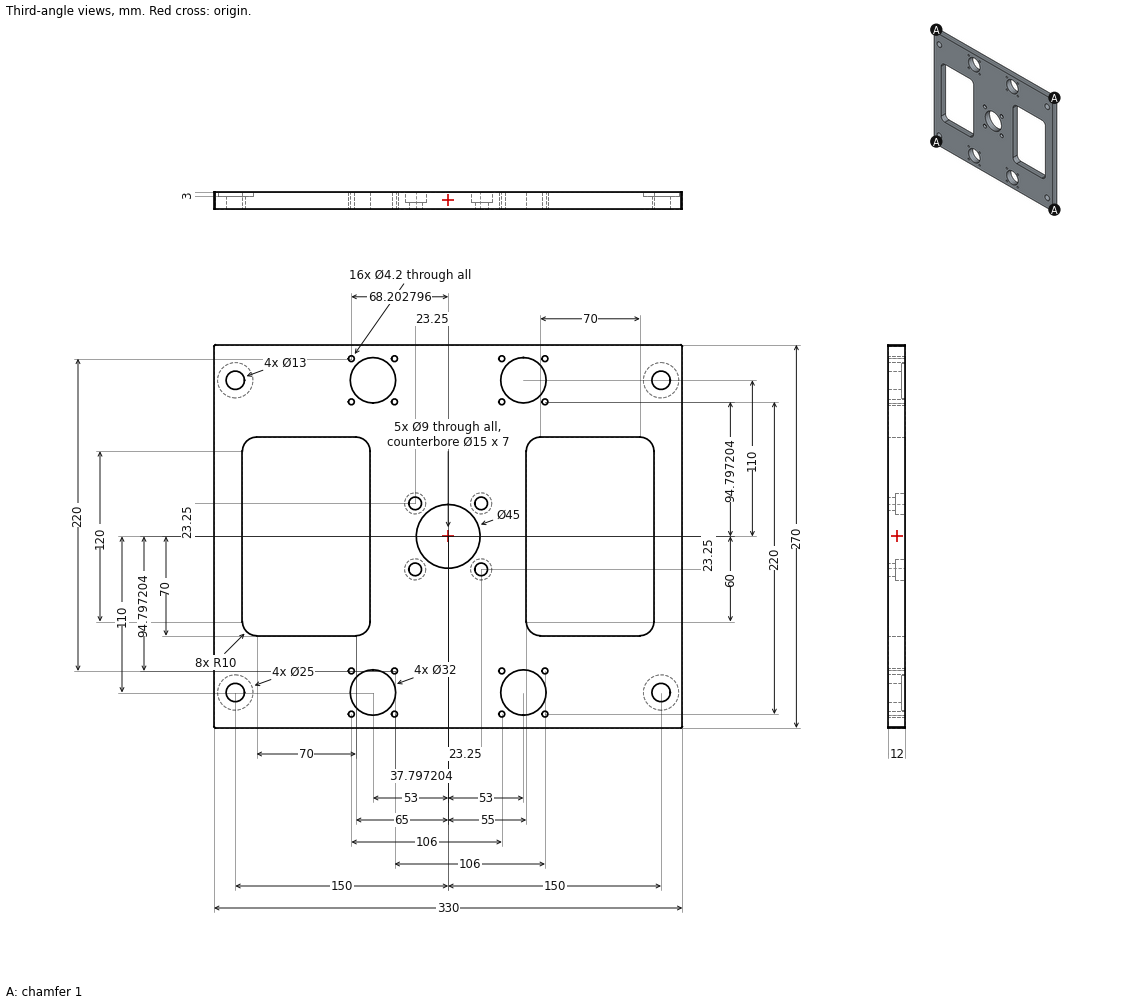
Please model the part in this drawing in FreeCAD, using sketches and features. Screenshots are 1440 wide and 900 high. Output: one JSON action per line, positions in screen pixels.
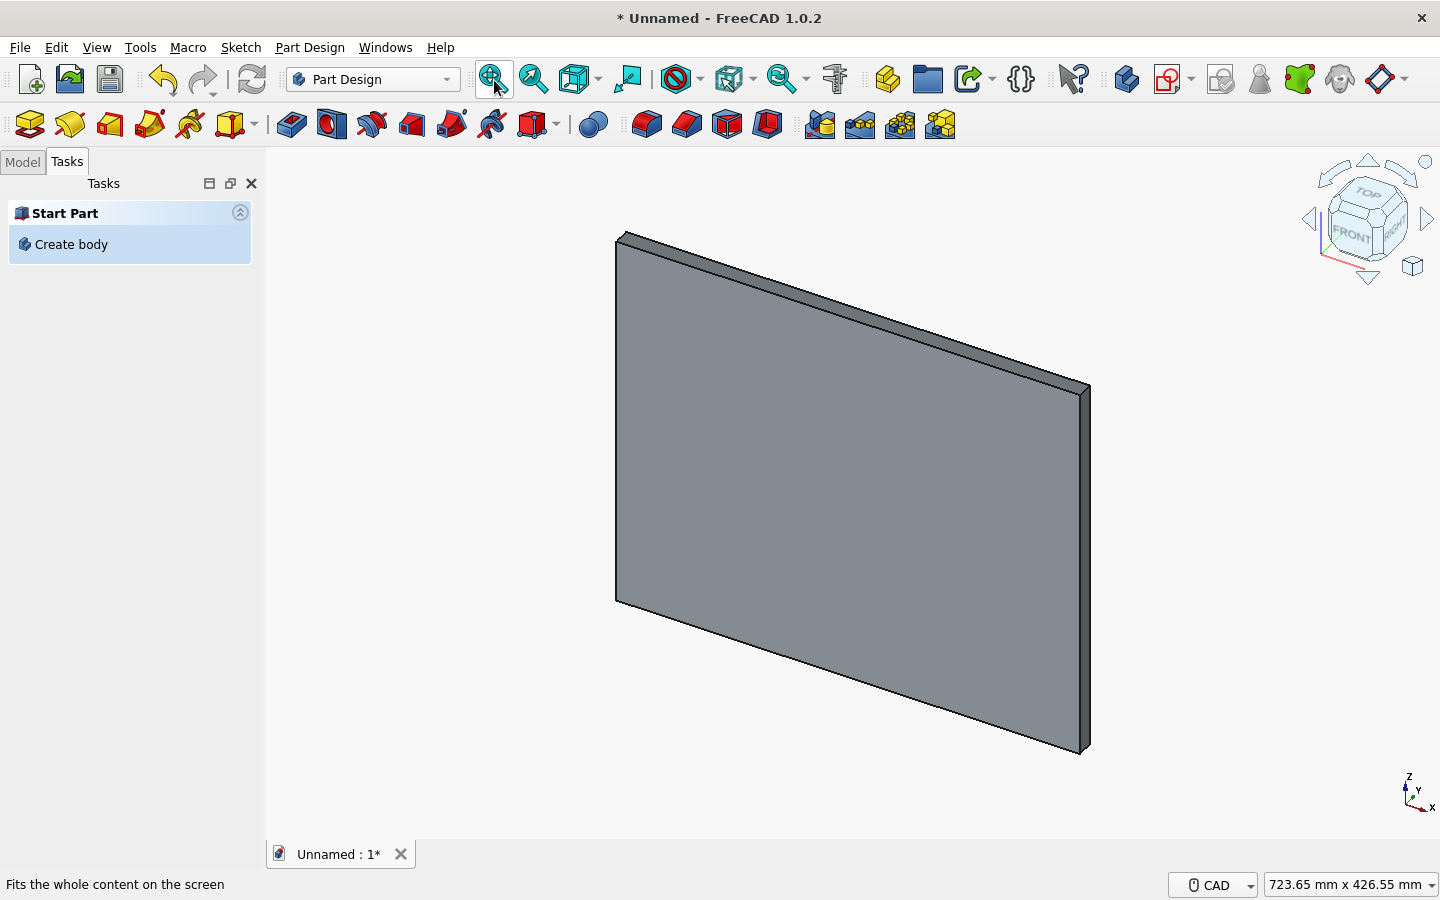
{"action": "key", "text": "4"}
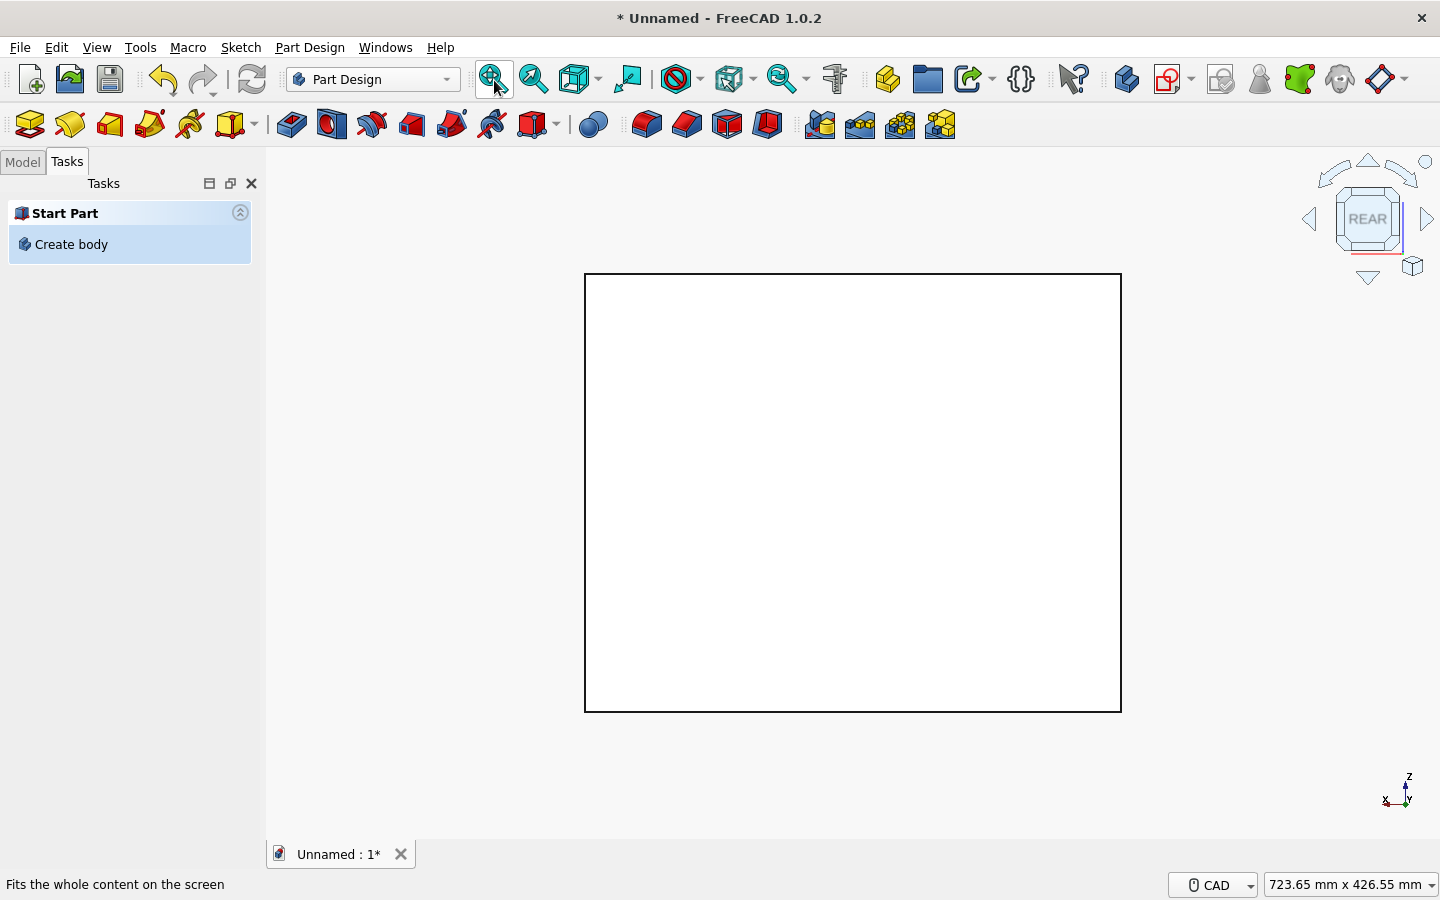
{"action": "left_click", "coordinate": [853, 492]}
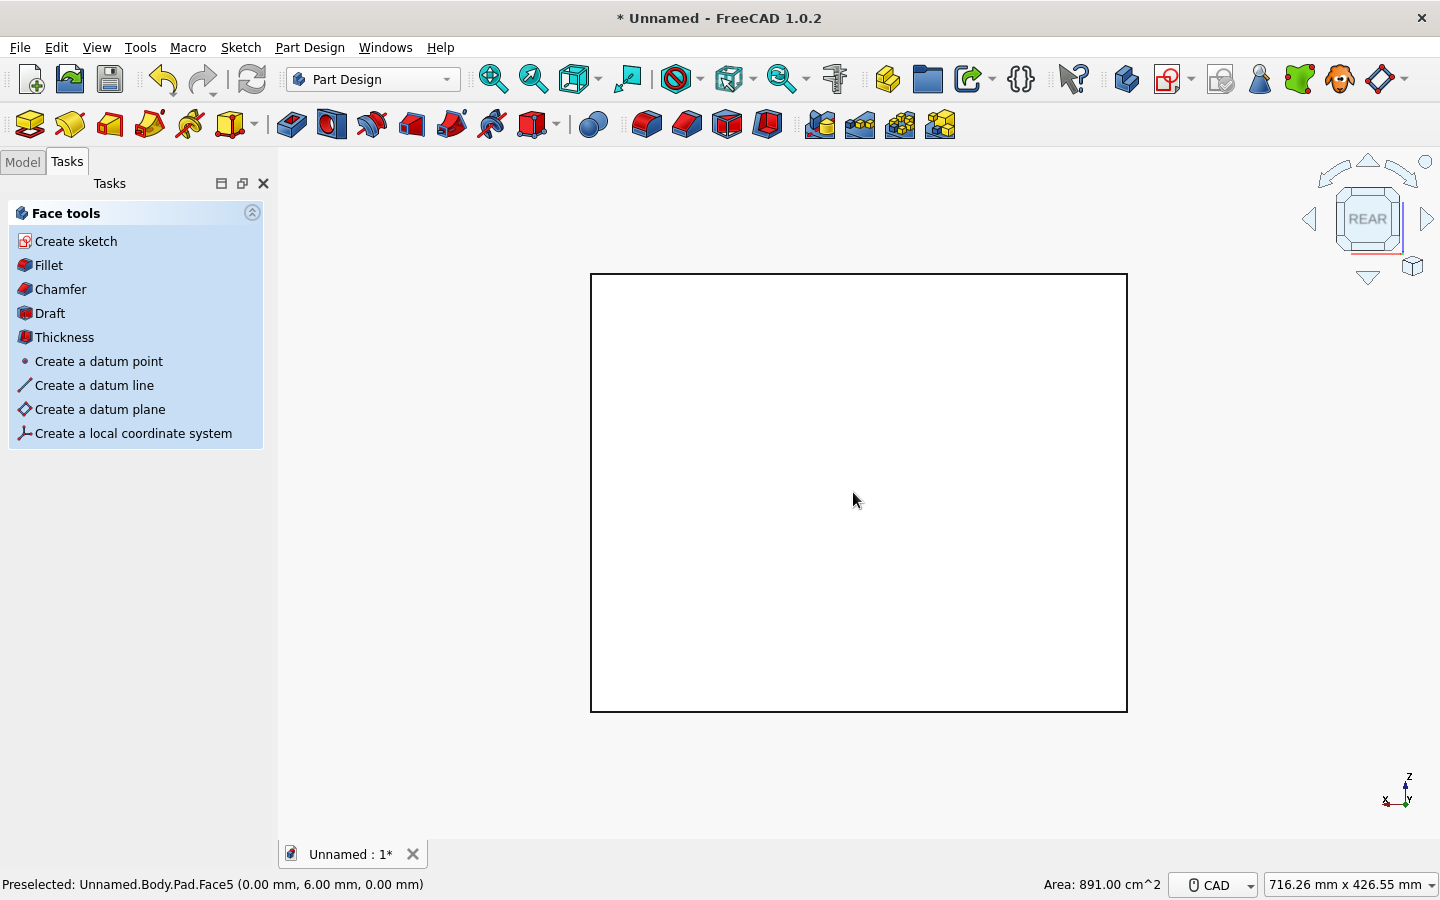
{"action": "left_click", "coordinate": [1168, 80]}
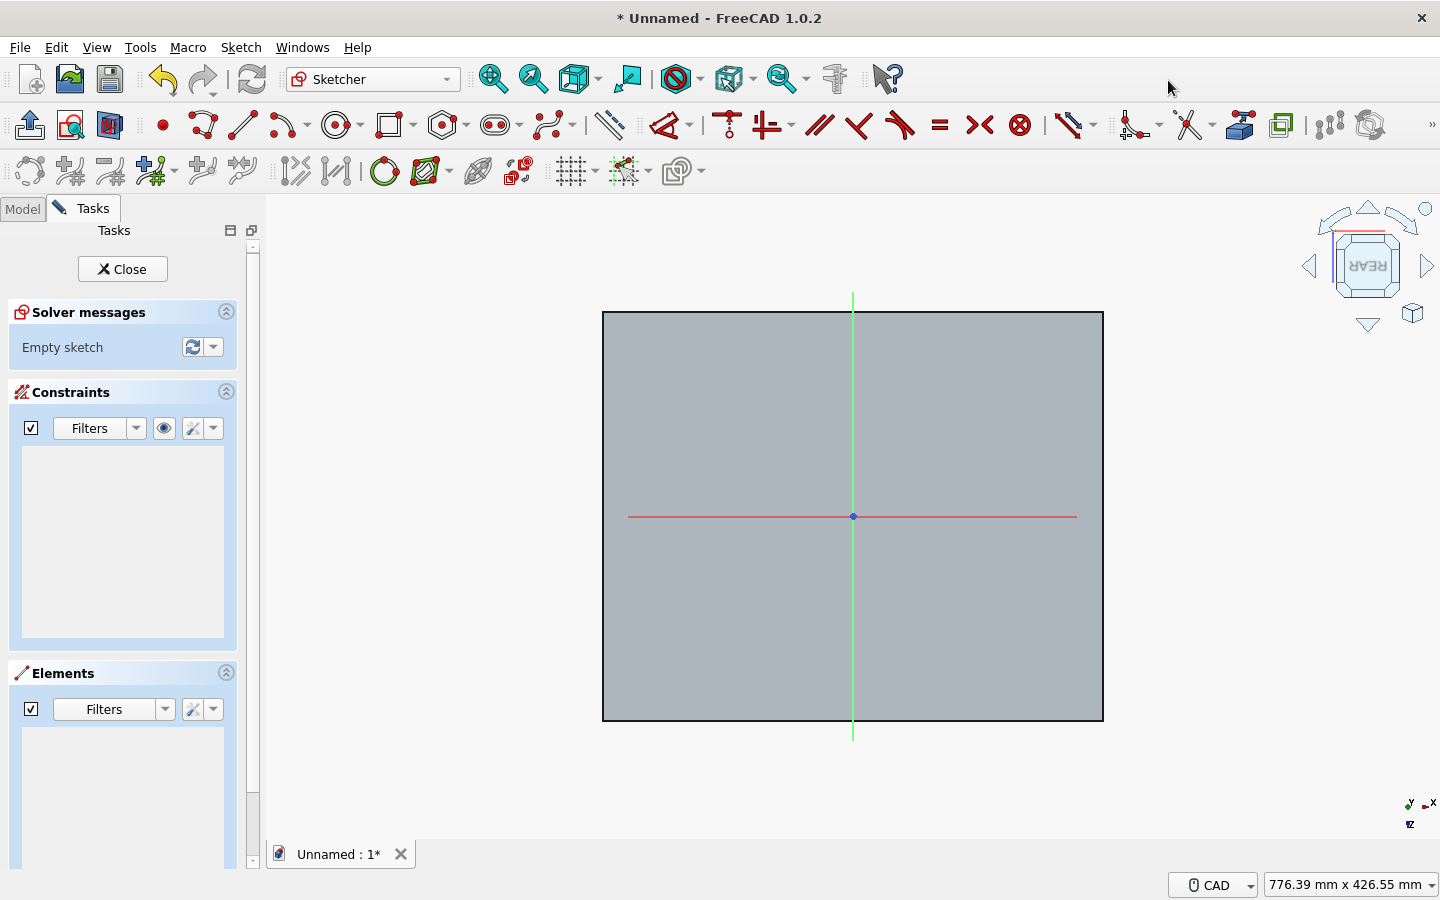
{"action": "left_click", "coordinate": [336, 126]}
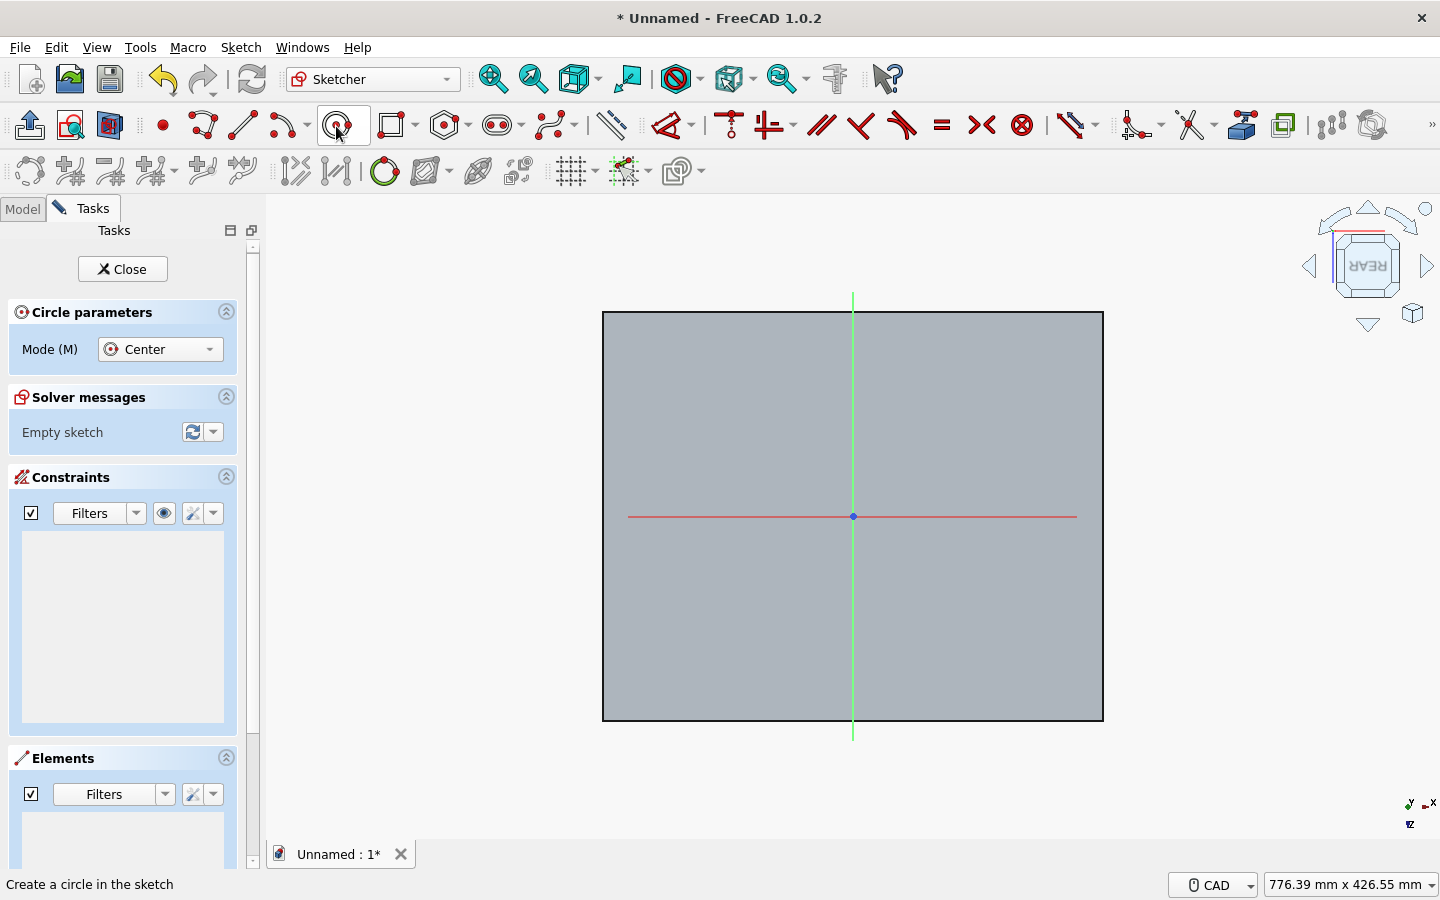
{"action": "left_click", "coordinate": [773, 350]}
{"action": "mouse_move", "coordinate": [790, 333]}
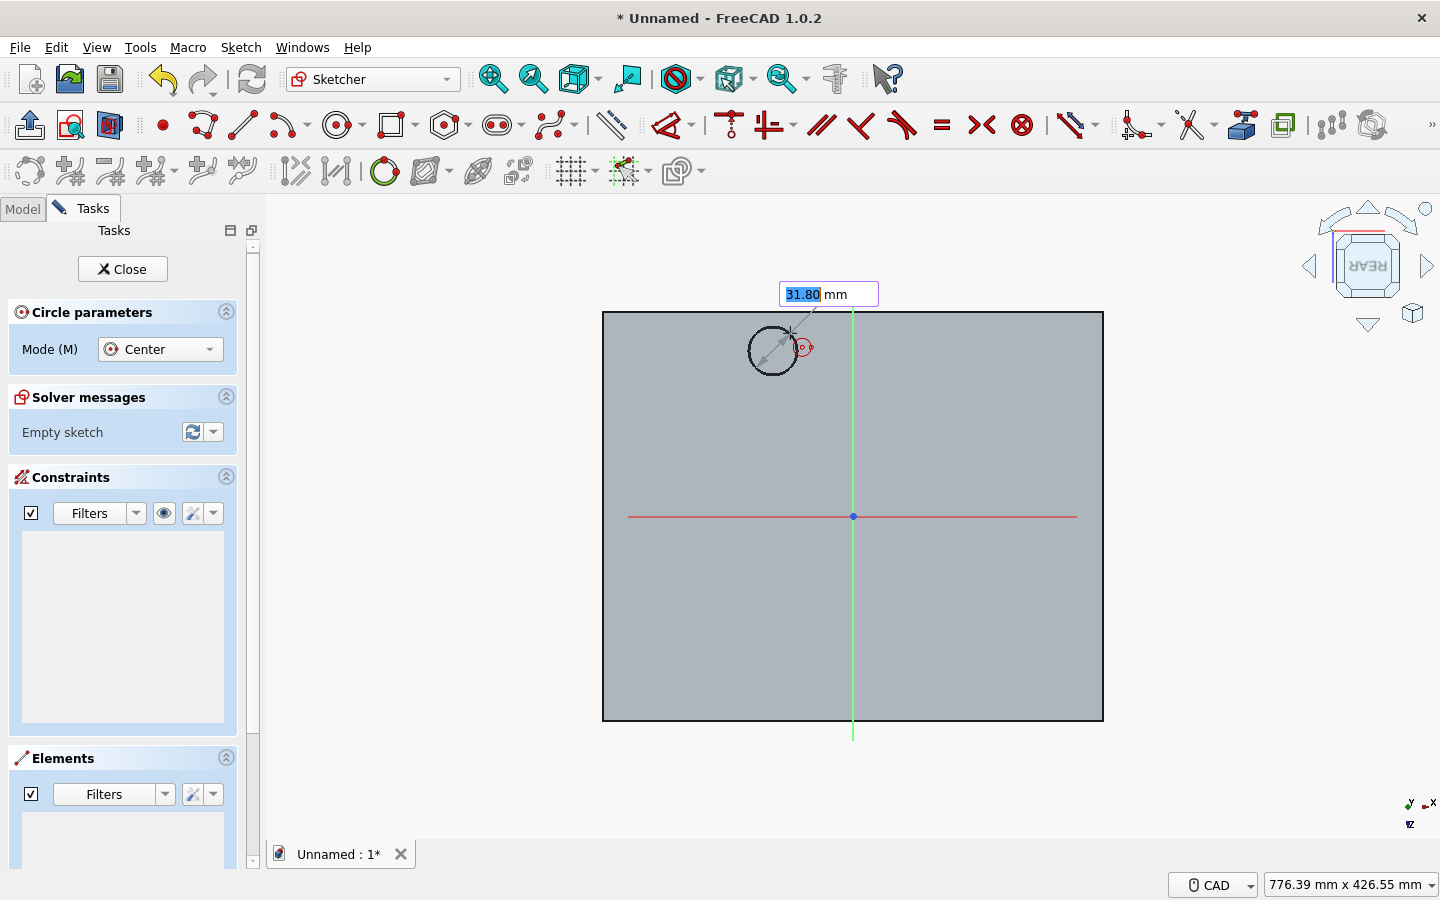
{"action": "type", "text": "32"}
{"action": "key", "text": "Return"}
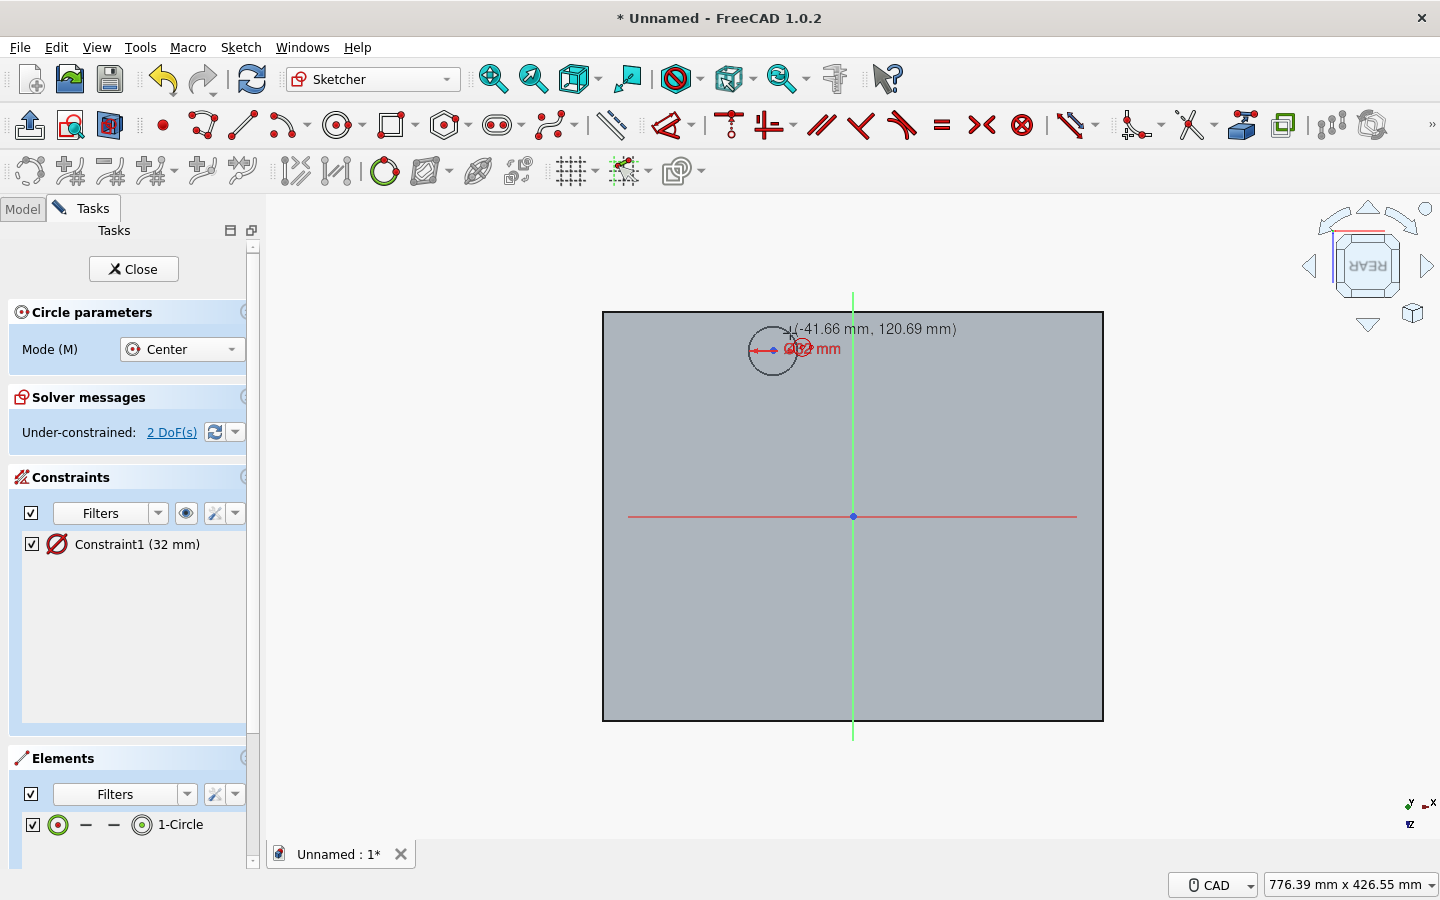
{"action": "left_click", "coordinate": [933, 350]}
{"action": "mouse_move", "coordinate": [950, 333]}